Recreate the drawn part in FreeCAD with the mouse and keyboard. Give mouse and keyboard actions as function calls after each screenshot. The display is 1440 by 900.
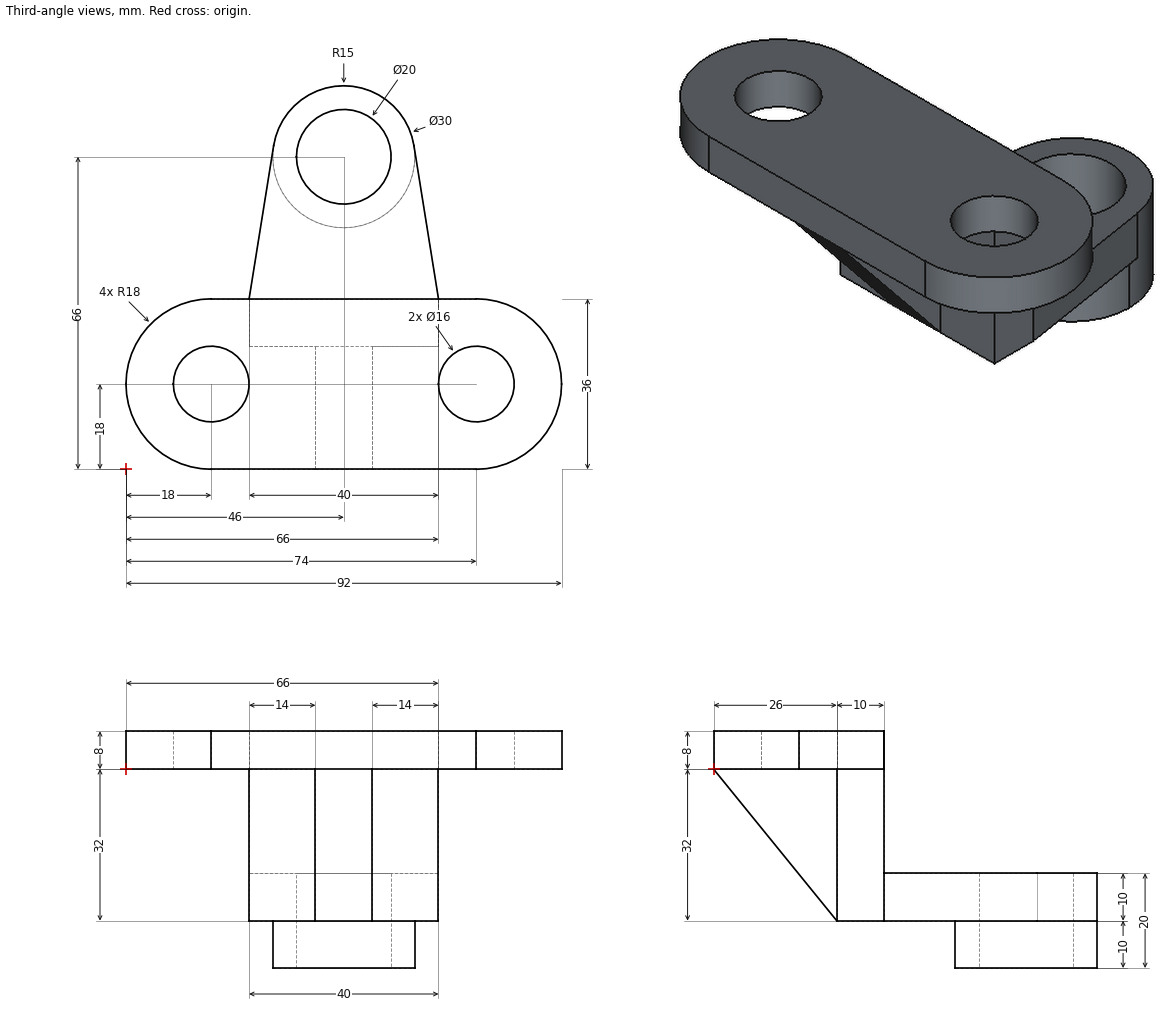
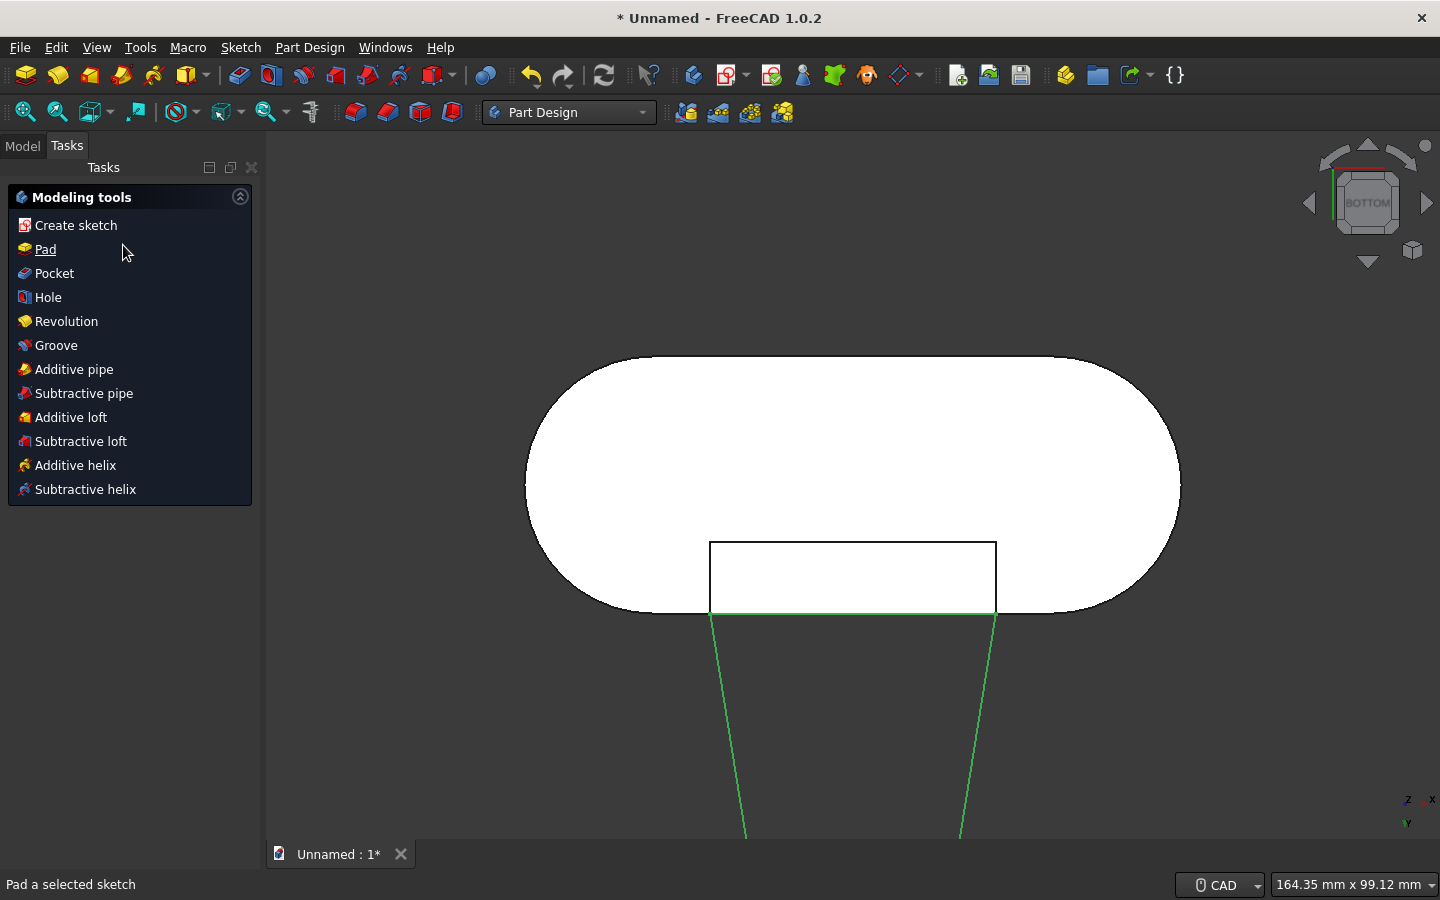
click(26, 76)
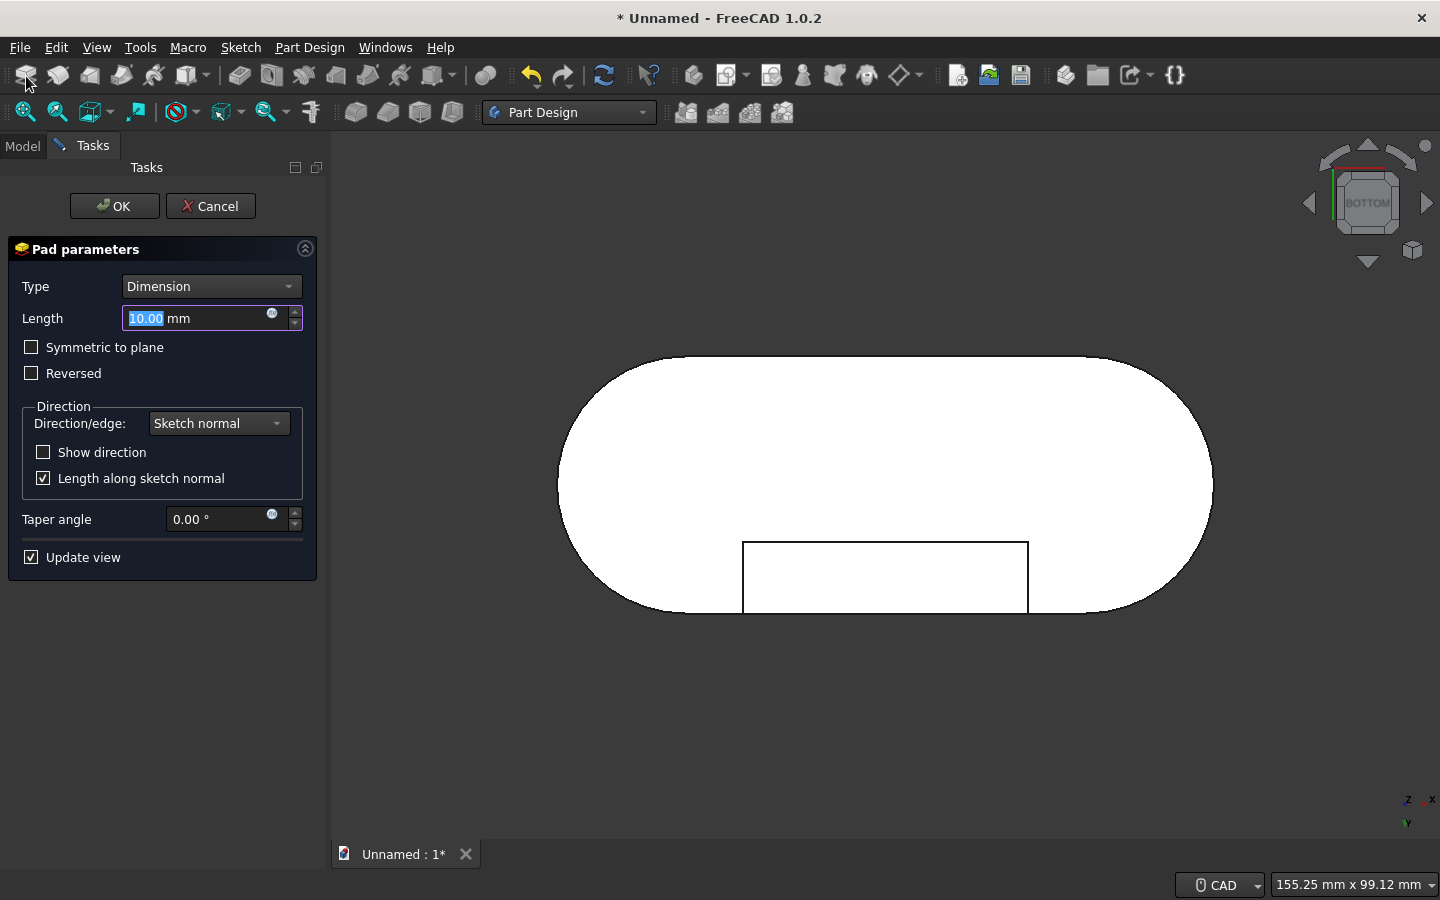
text(10)
key(Tab)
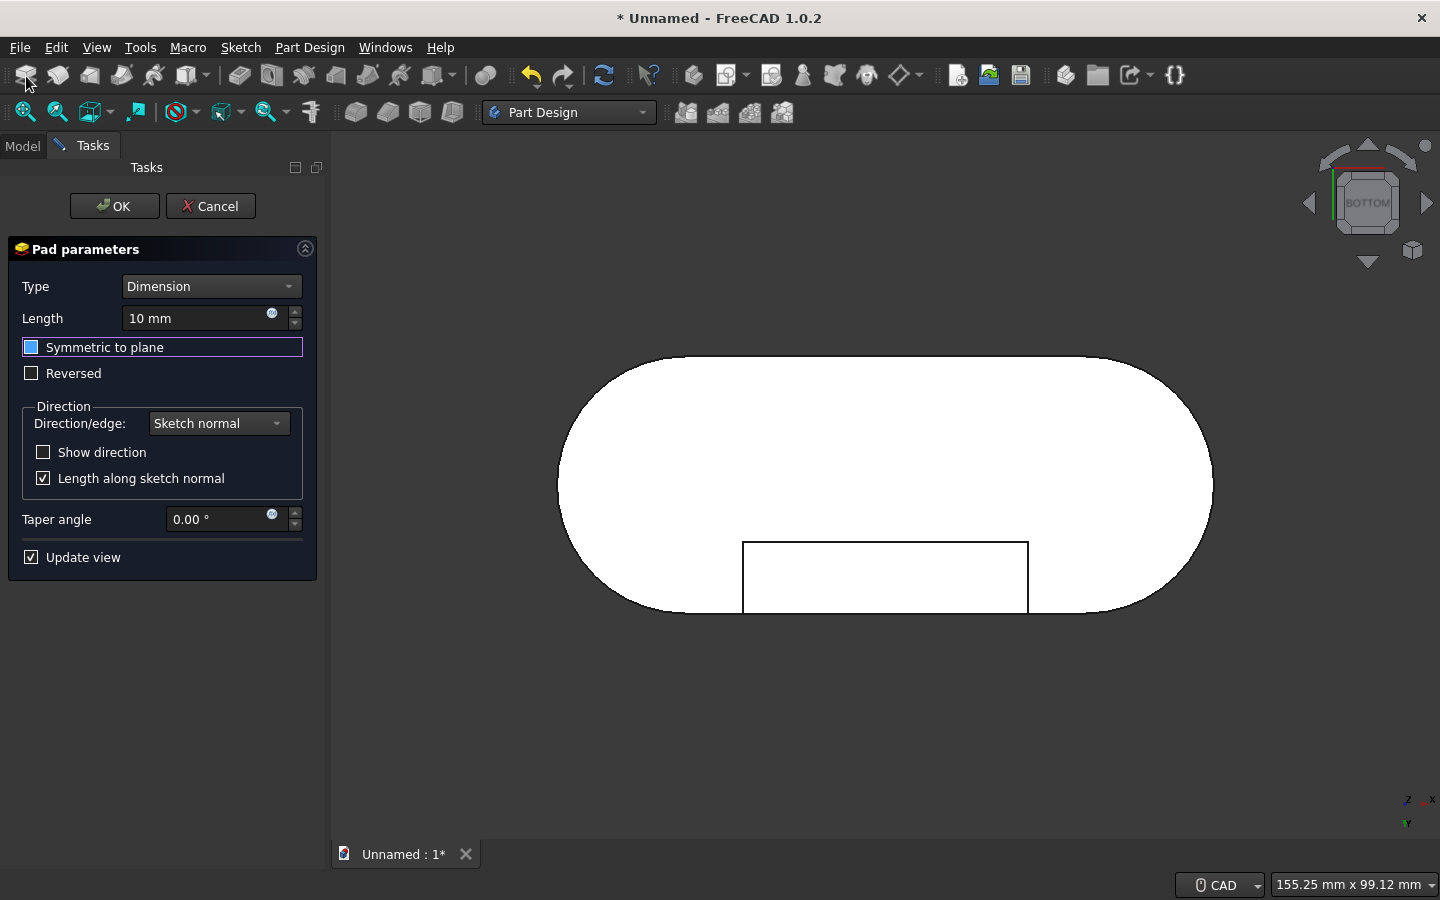
click(30, 373)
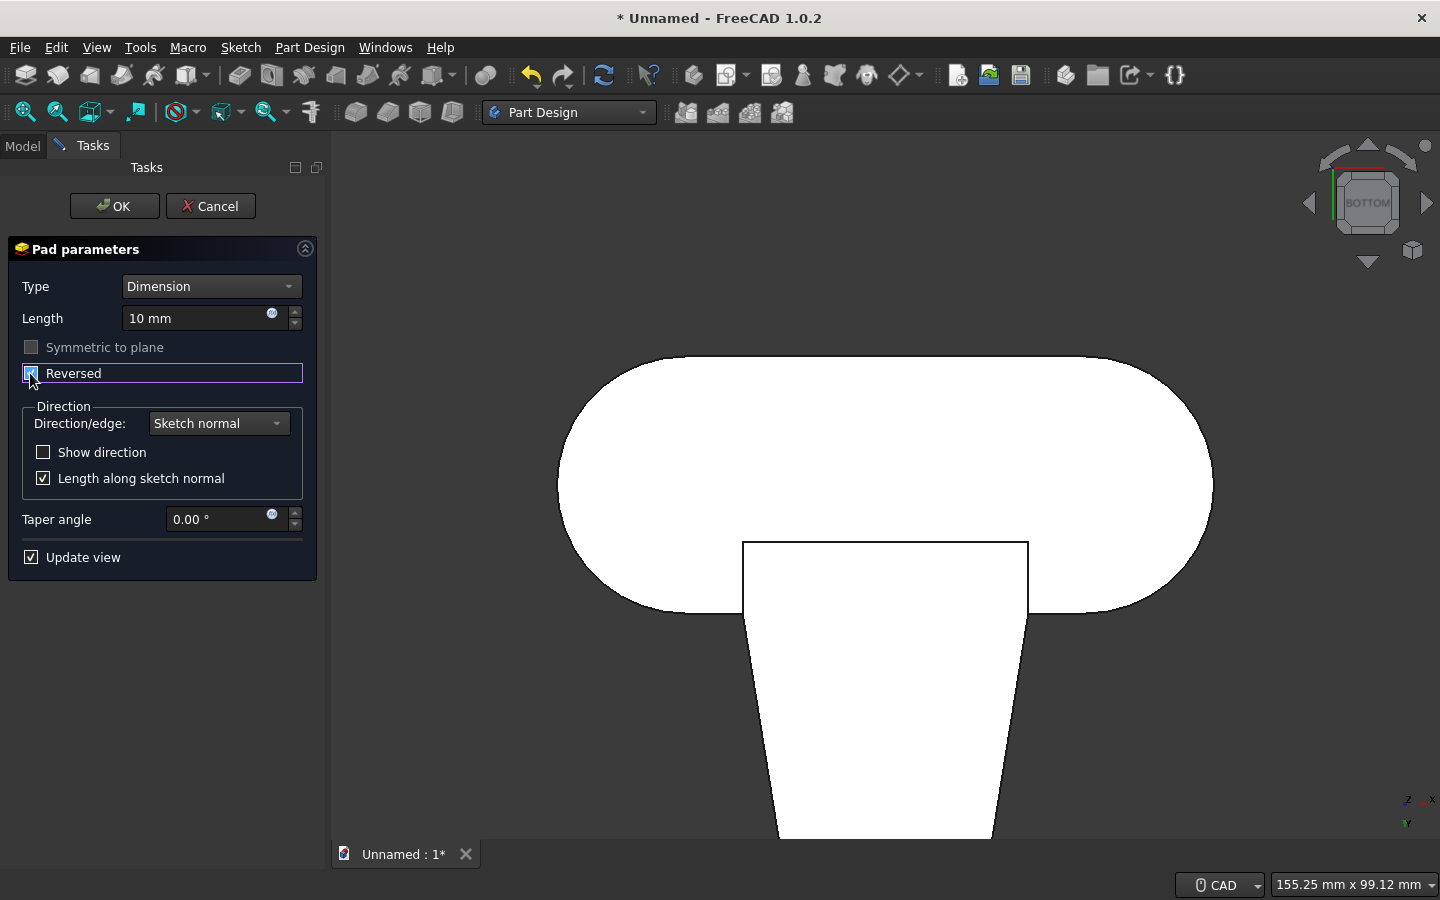
click(115, 206)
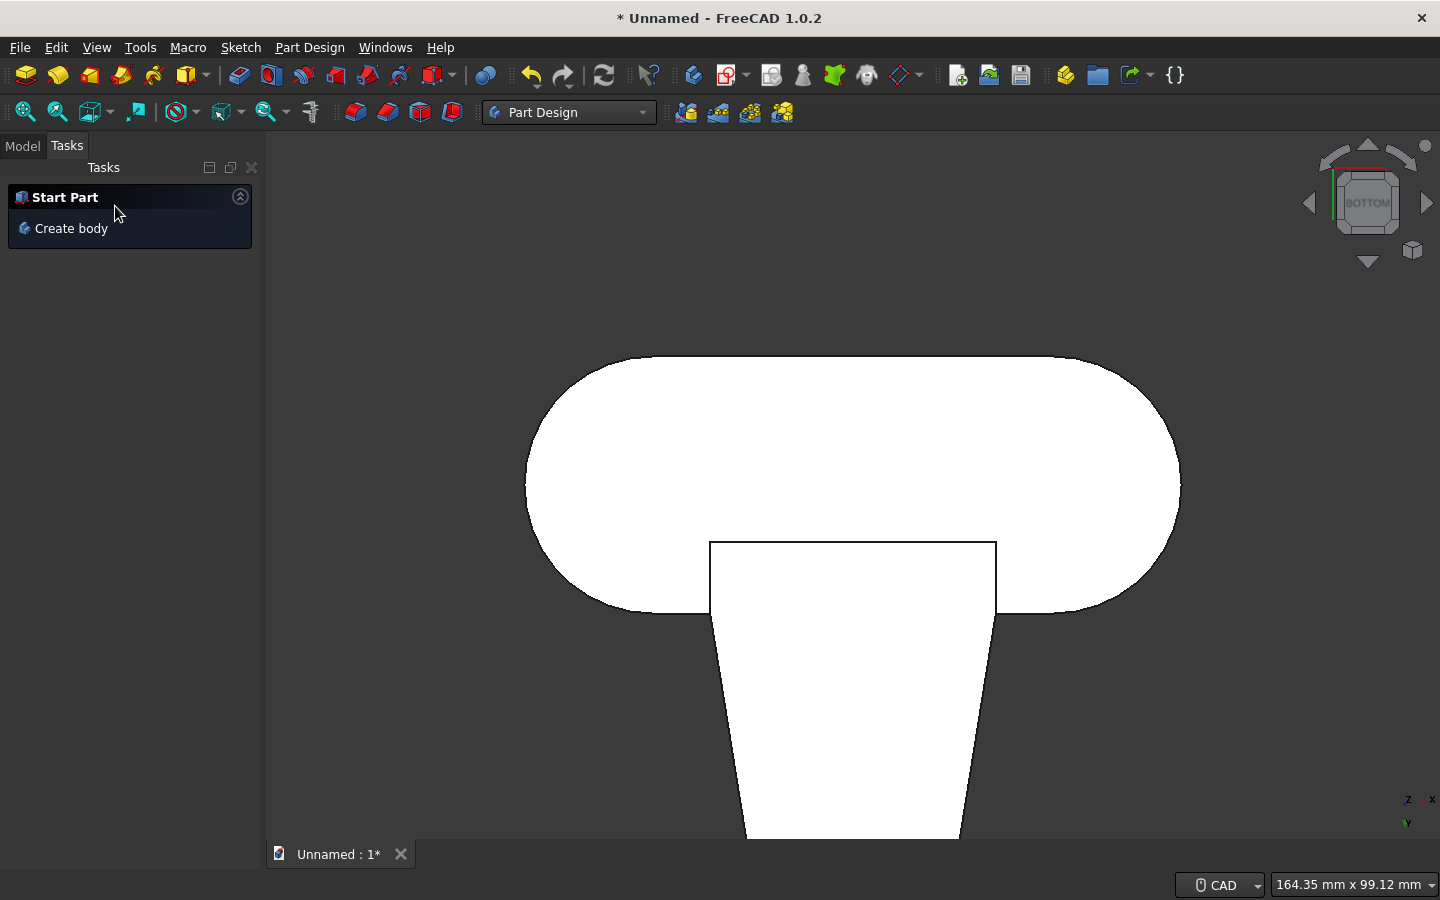
click(26, 112)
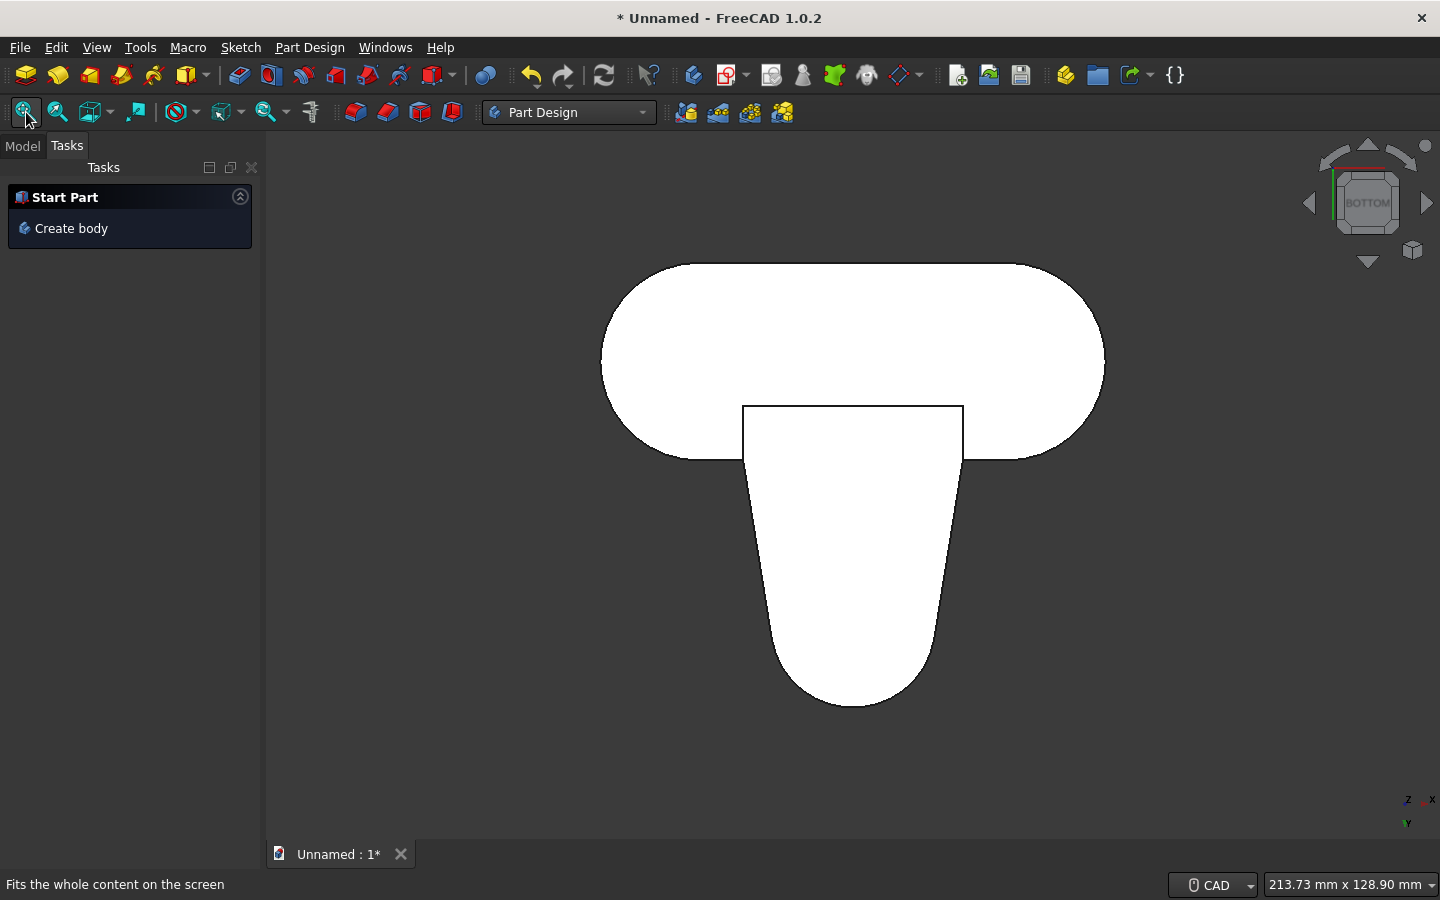
click(23, 145)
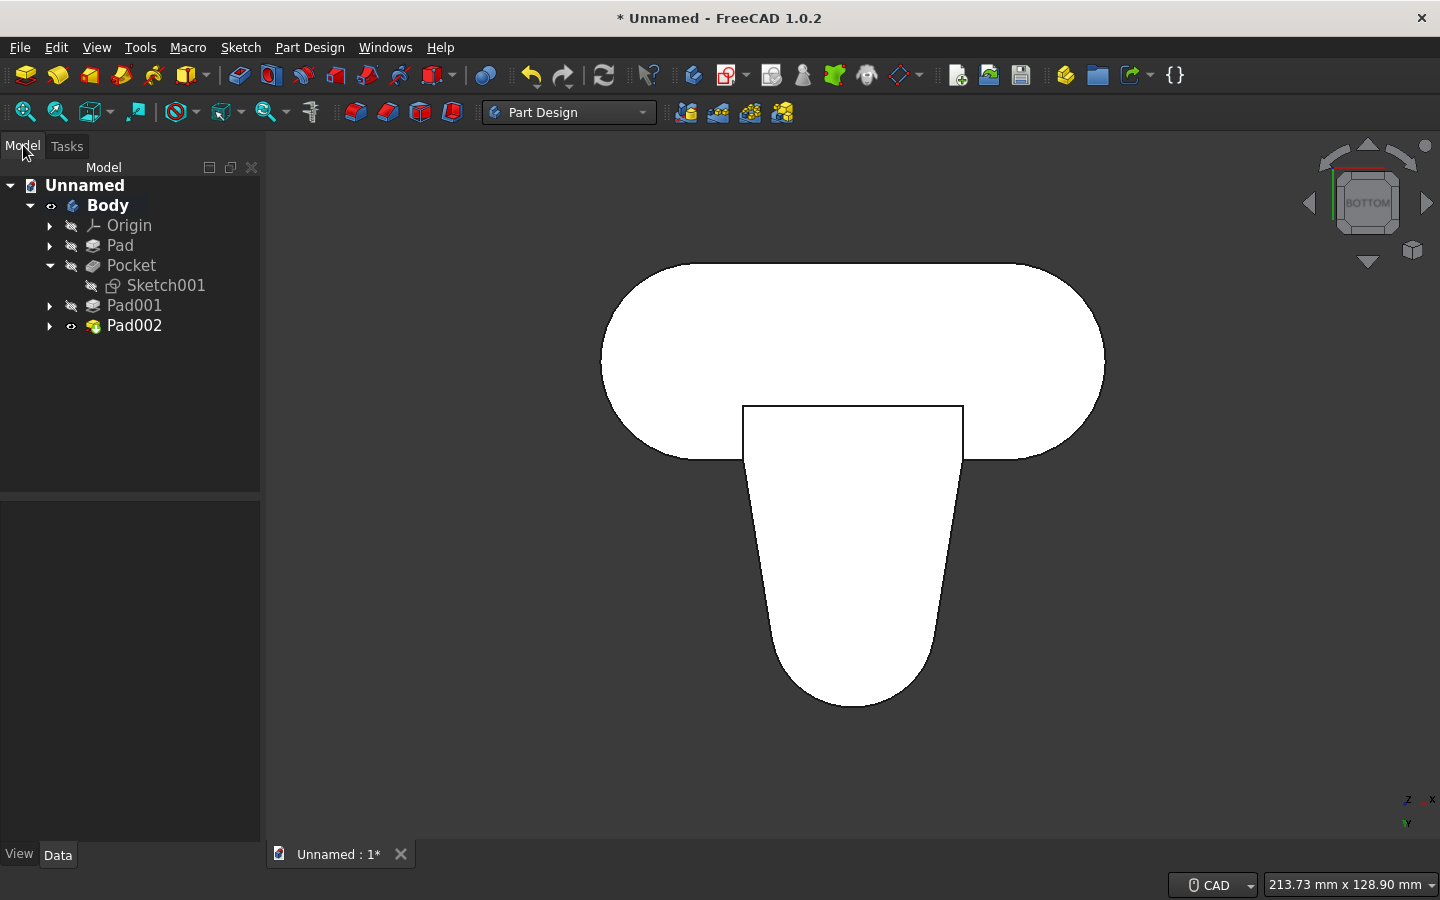
click(50, 226)